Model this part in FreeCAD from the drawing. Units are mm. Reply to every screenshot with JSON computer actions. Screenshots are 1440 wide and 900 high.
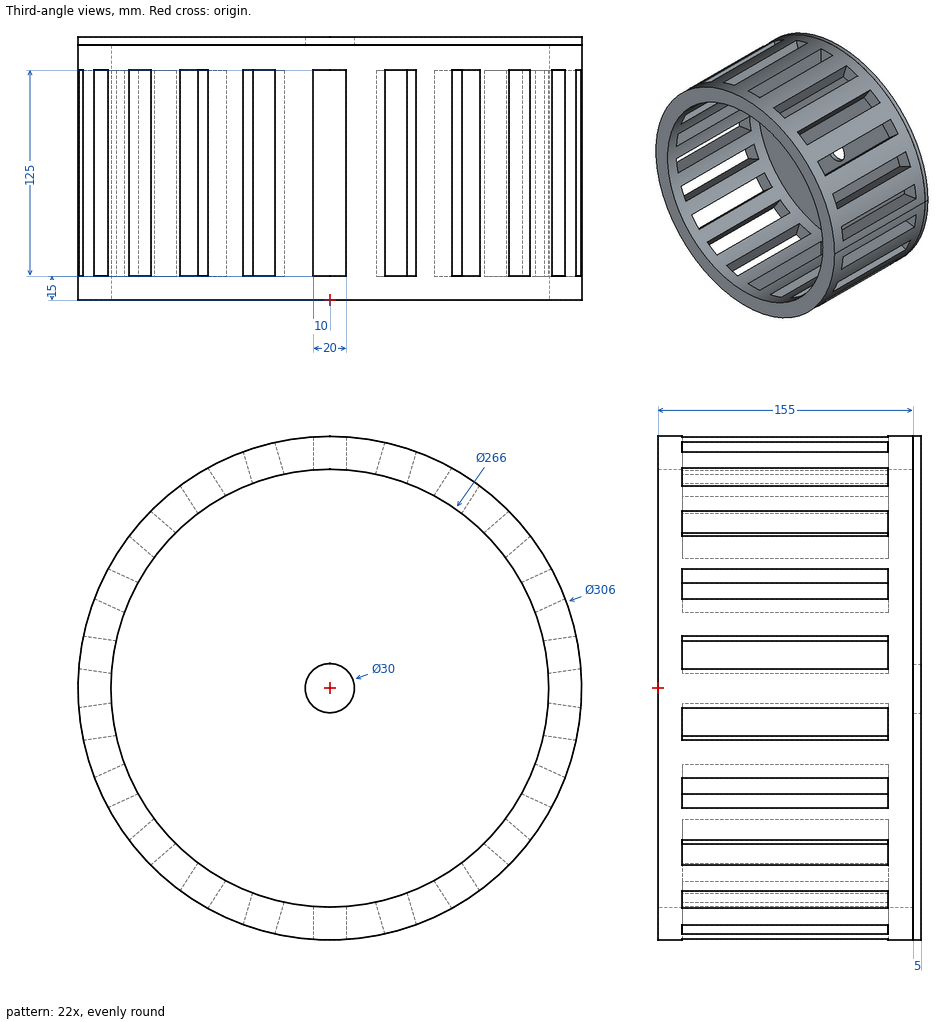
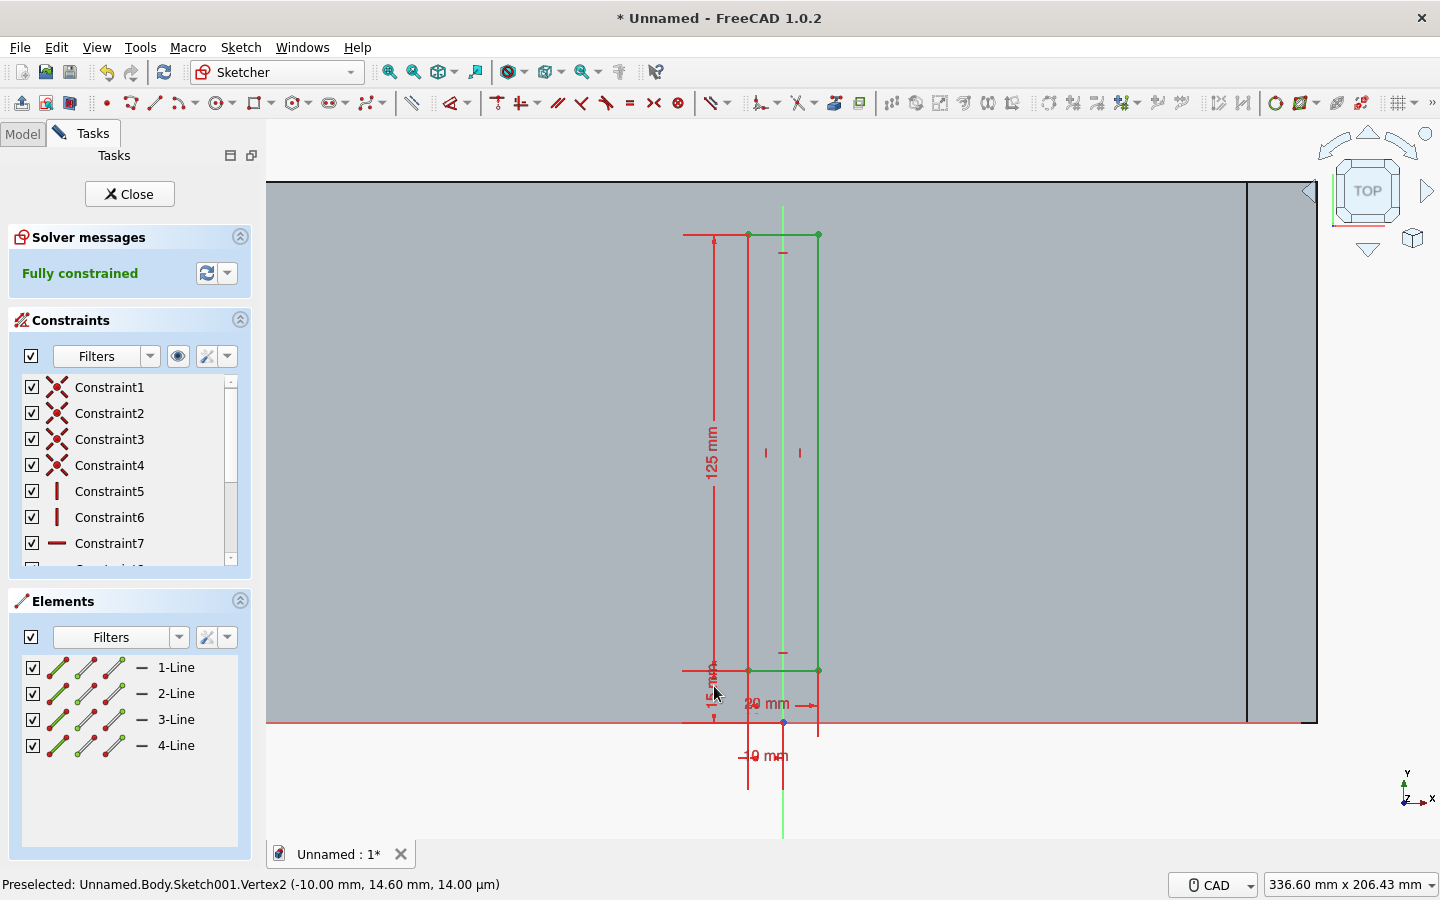
{"action": "left_click", "coordinate": [130, 194]}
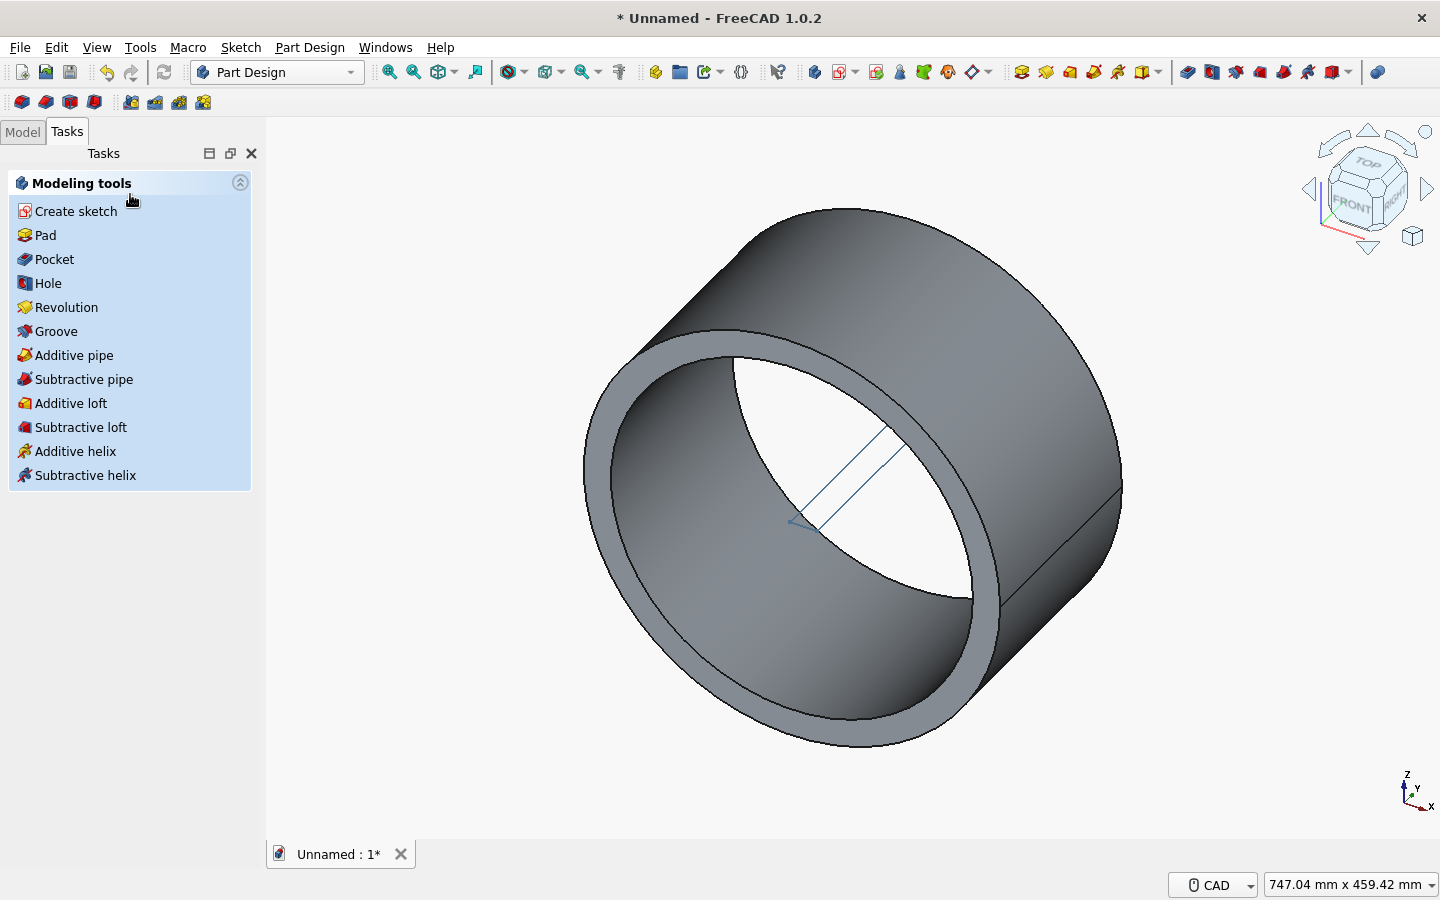
{"action": "left_click", "coordinate": [1188, 72]}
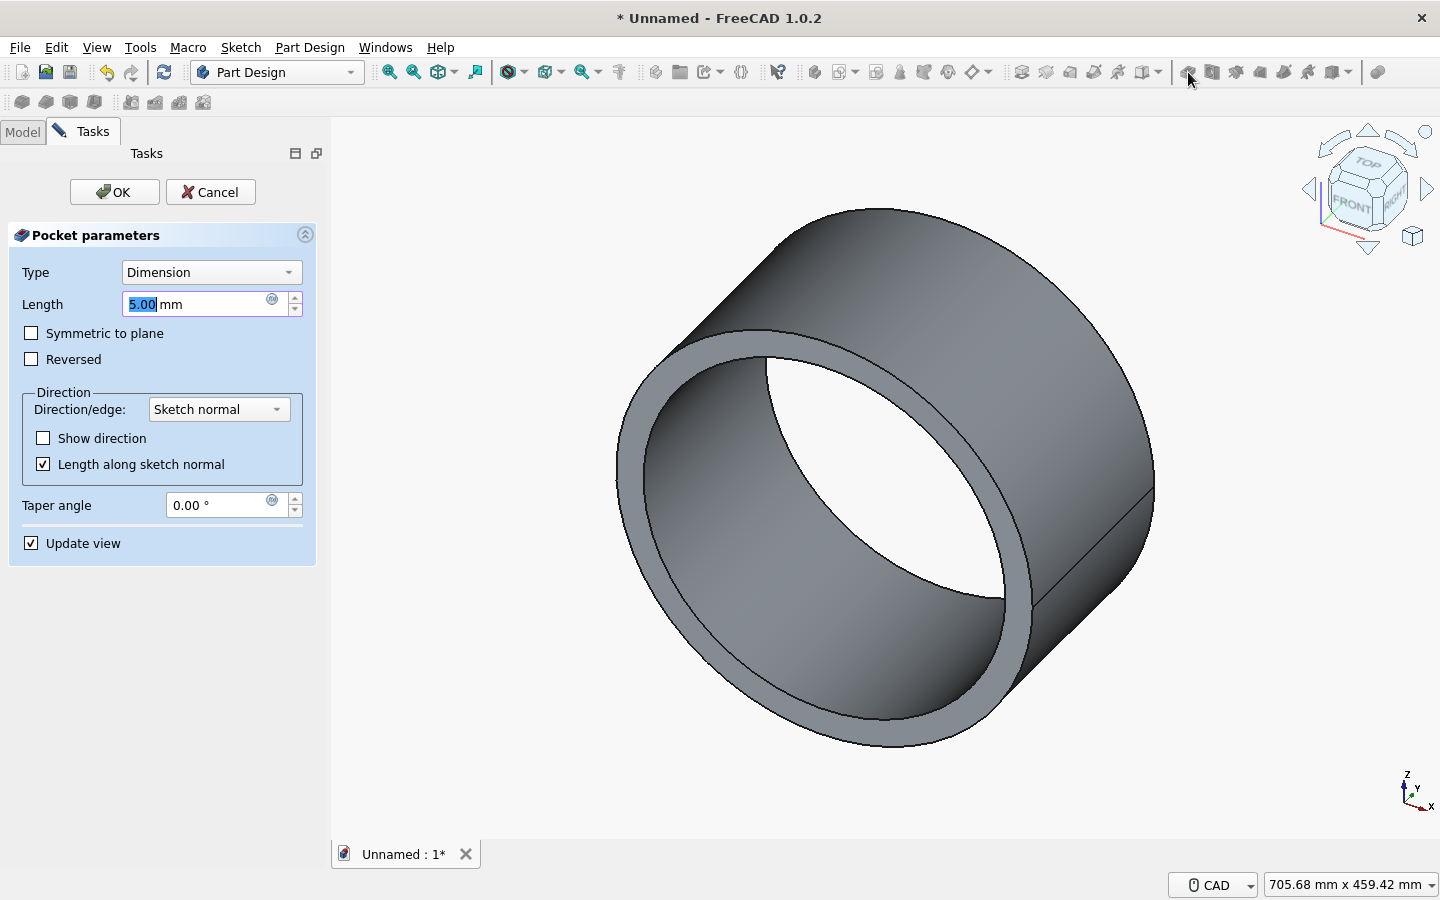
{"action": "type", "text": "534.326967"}
{"action": "key", "text": "Tab"}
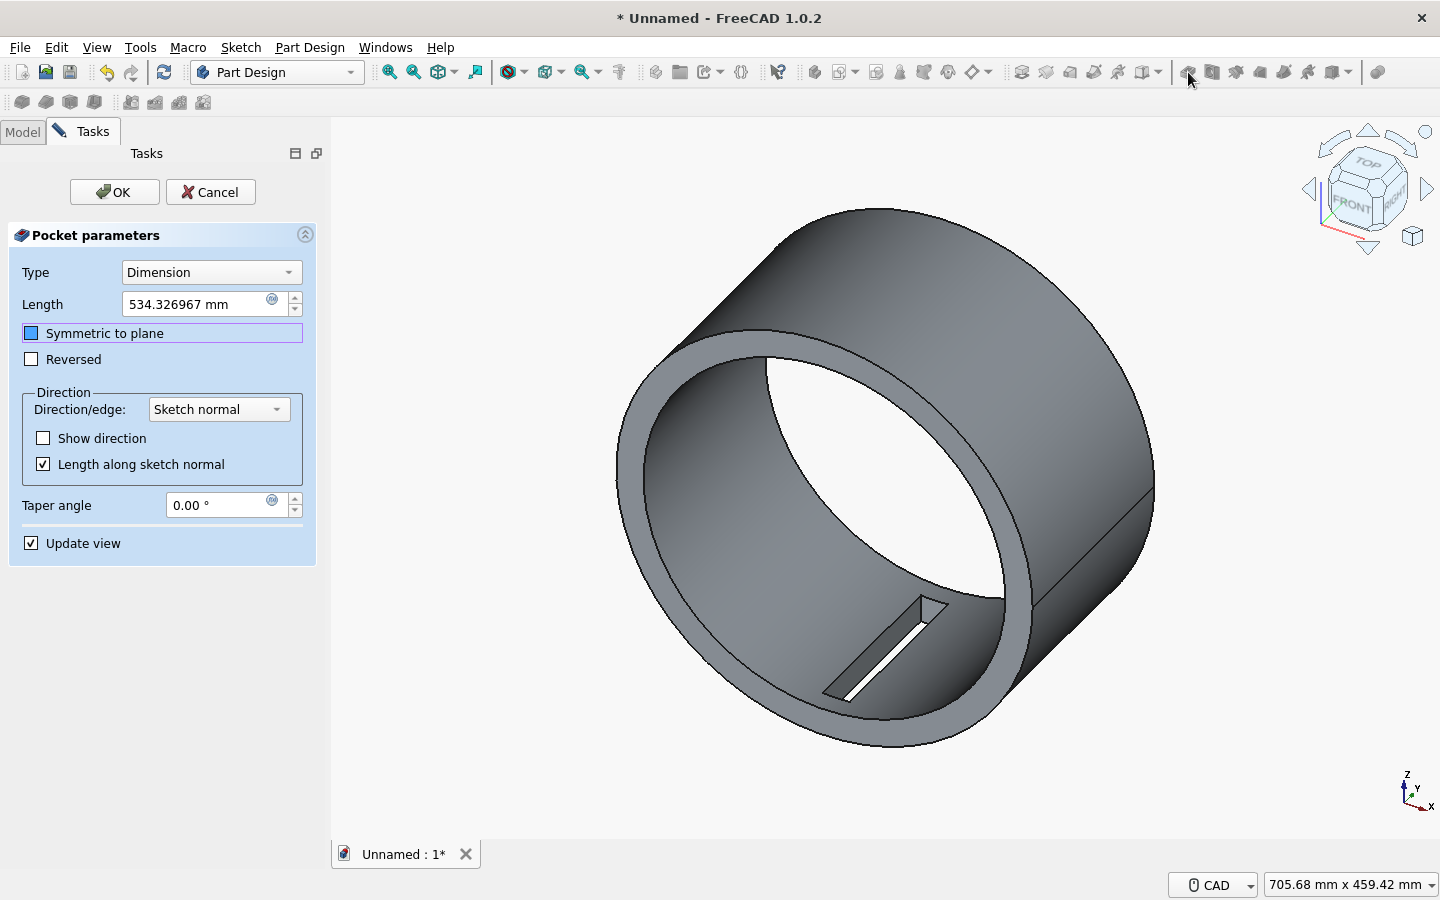
{"action": "left_click", "coordinate": [30, 333]}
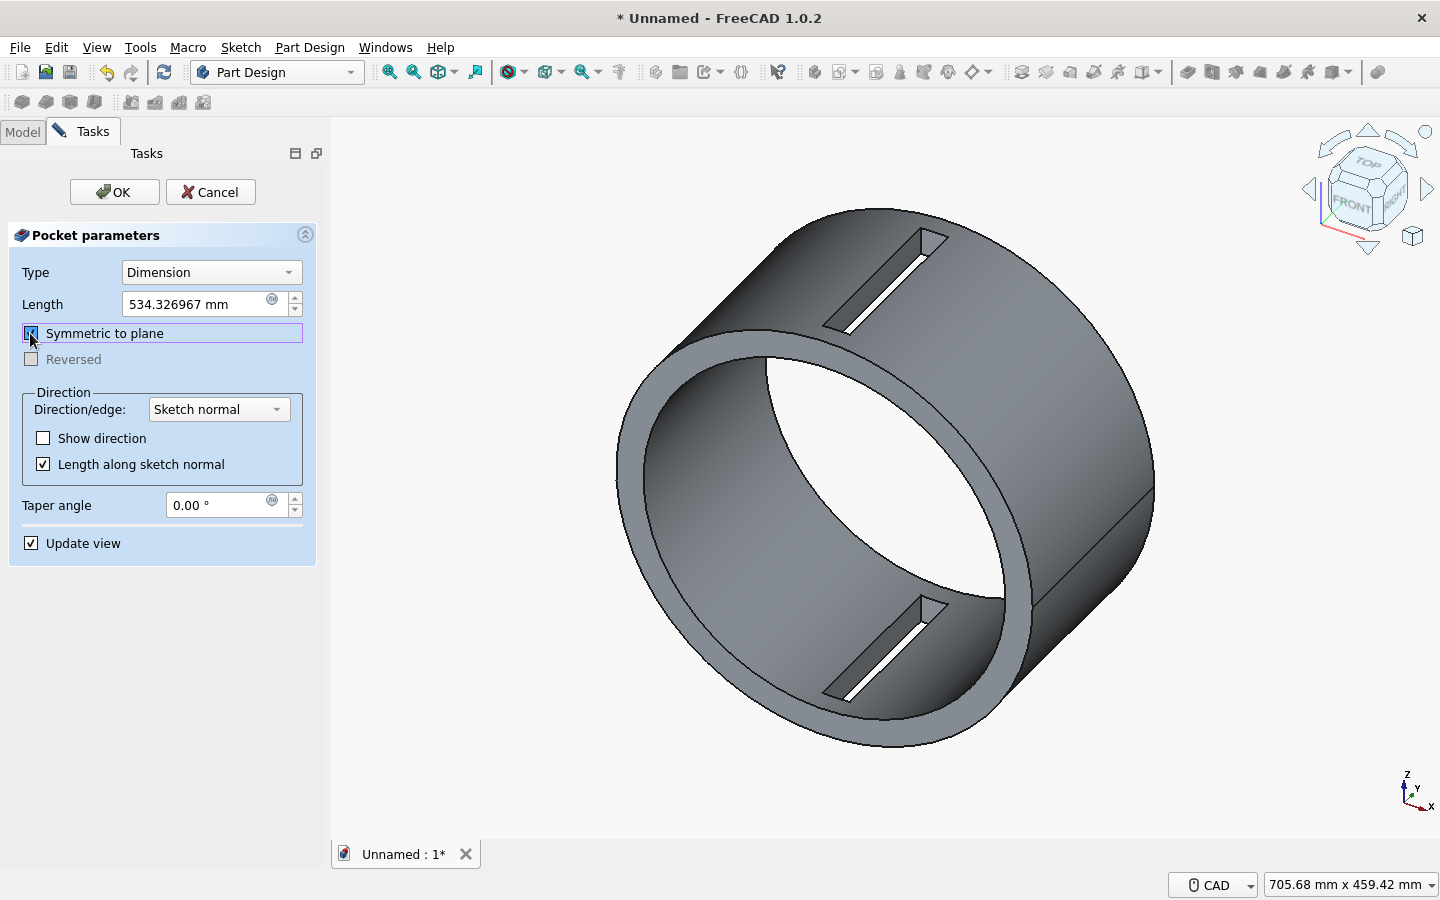
{"action": "left_click", "coordinate": [115, 192]}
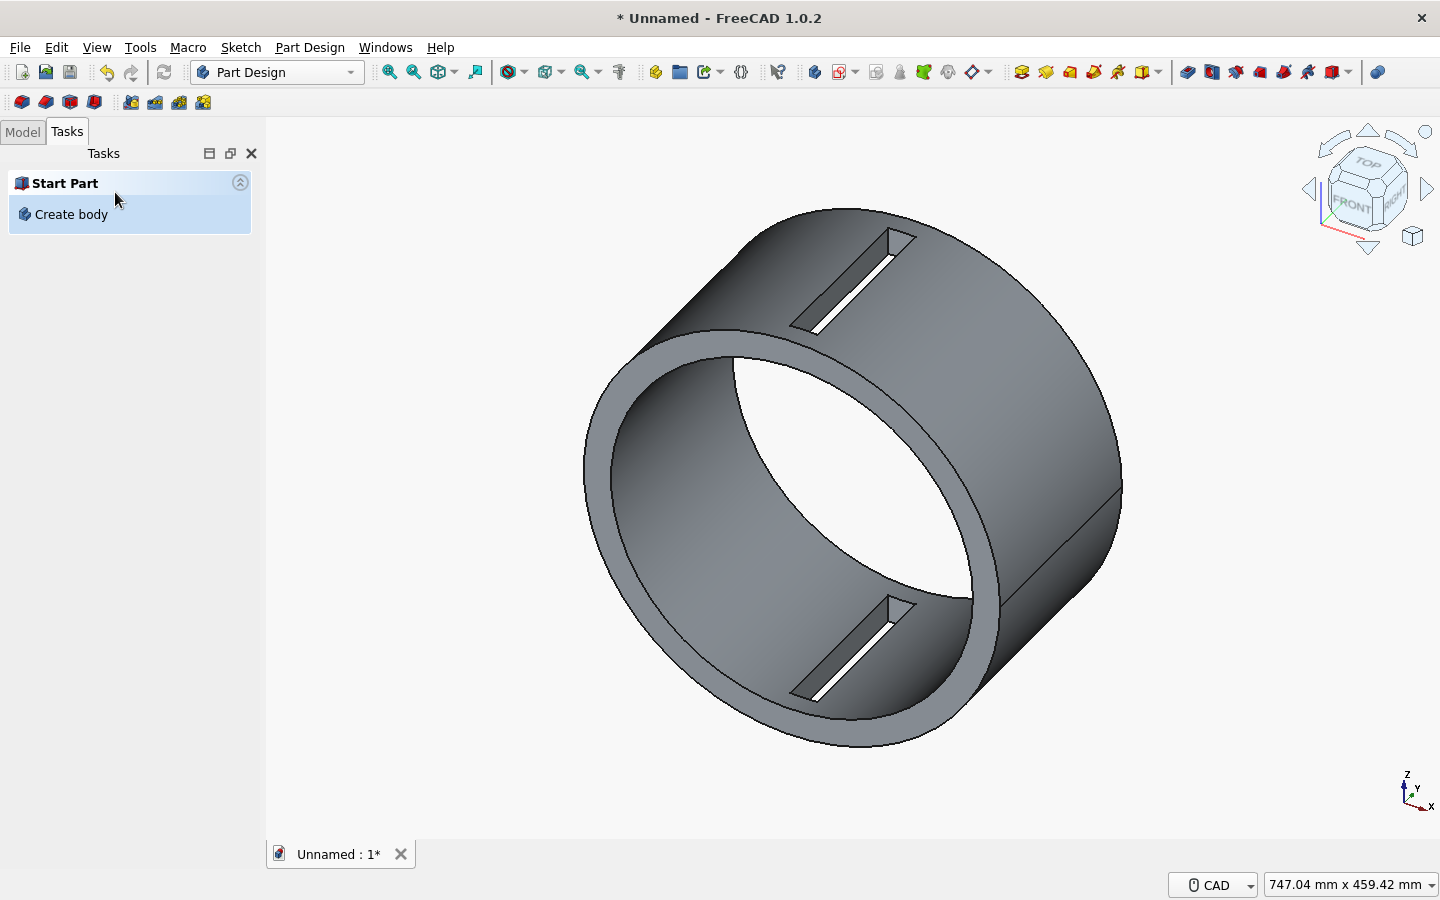
{"action": "left_click", "coordinate": [23, 131]}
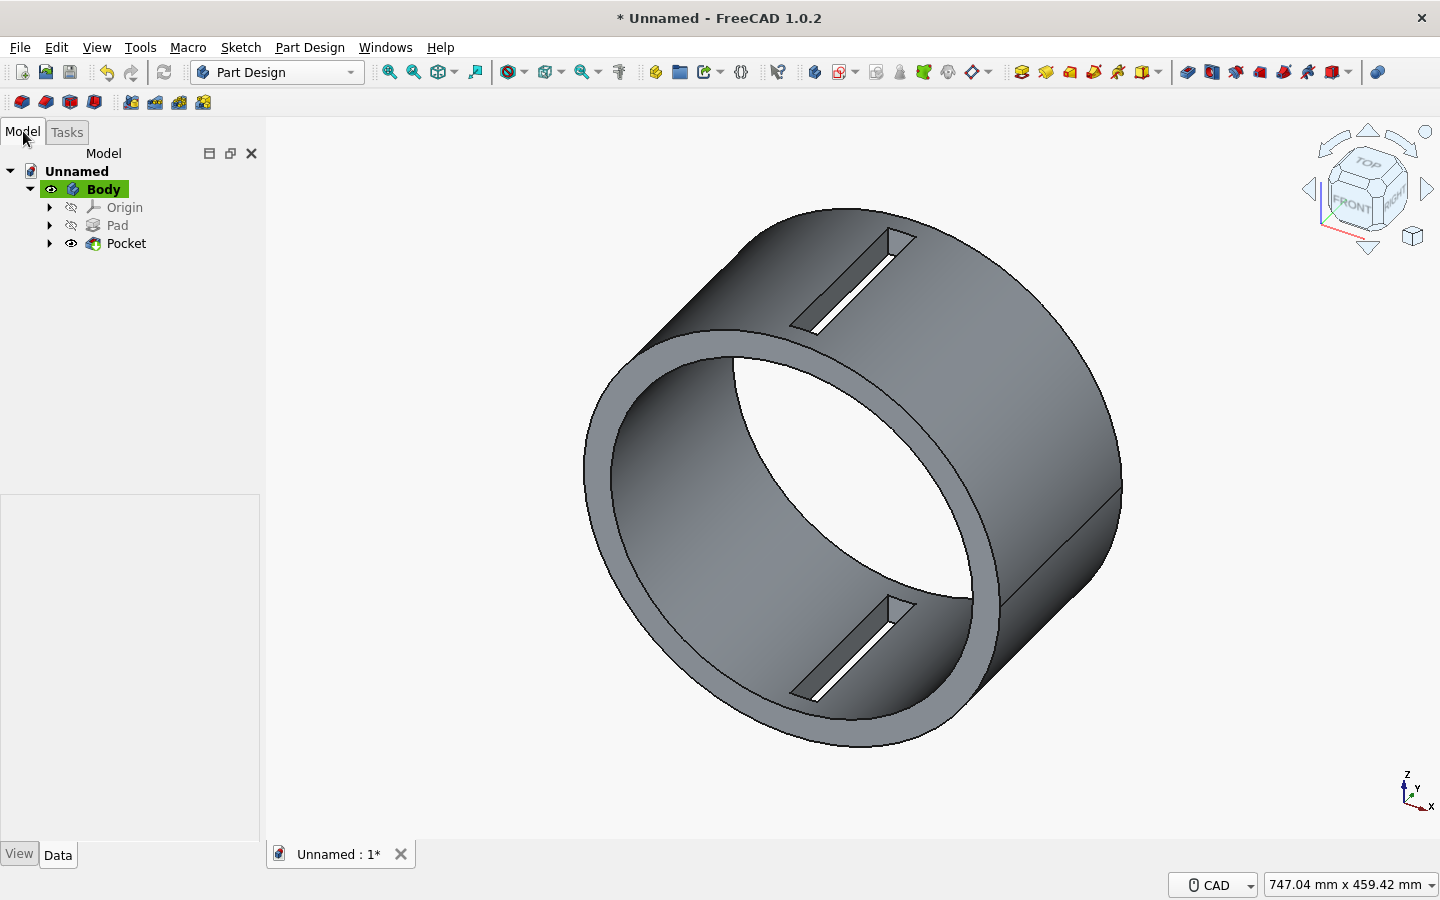
{"action": "left_click", "coordinate": [116, 243]}